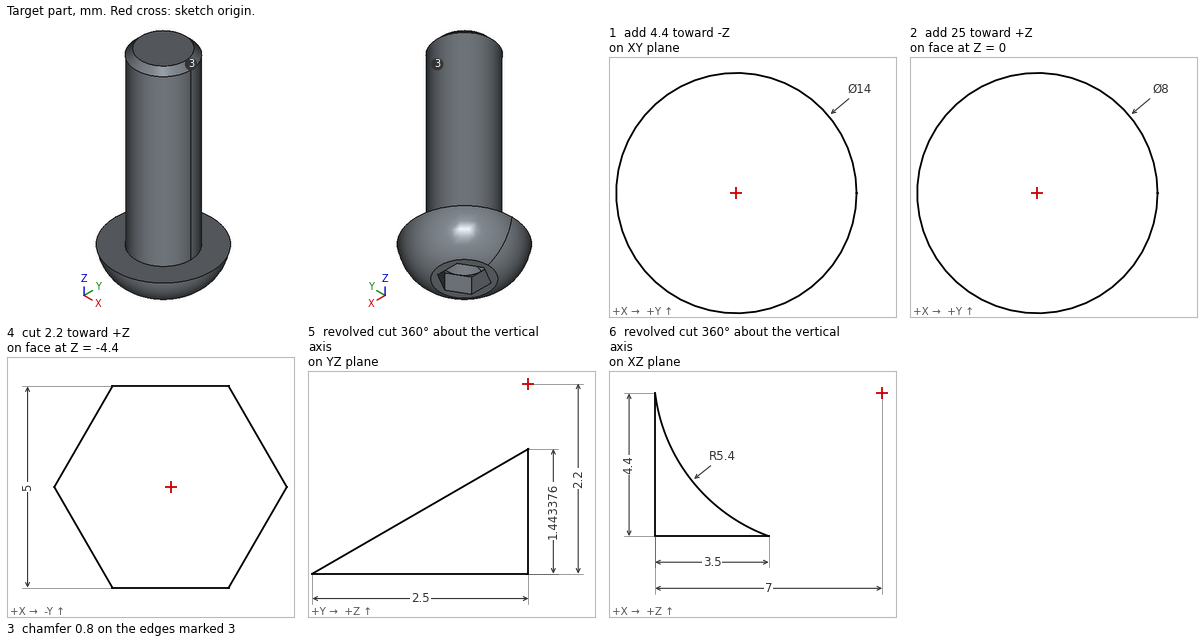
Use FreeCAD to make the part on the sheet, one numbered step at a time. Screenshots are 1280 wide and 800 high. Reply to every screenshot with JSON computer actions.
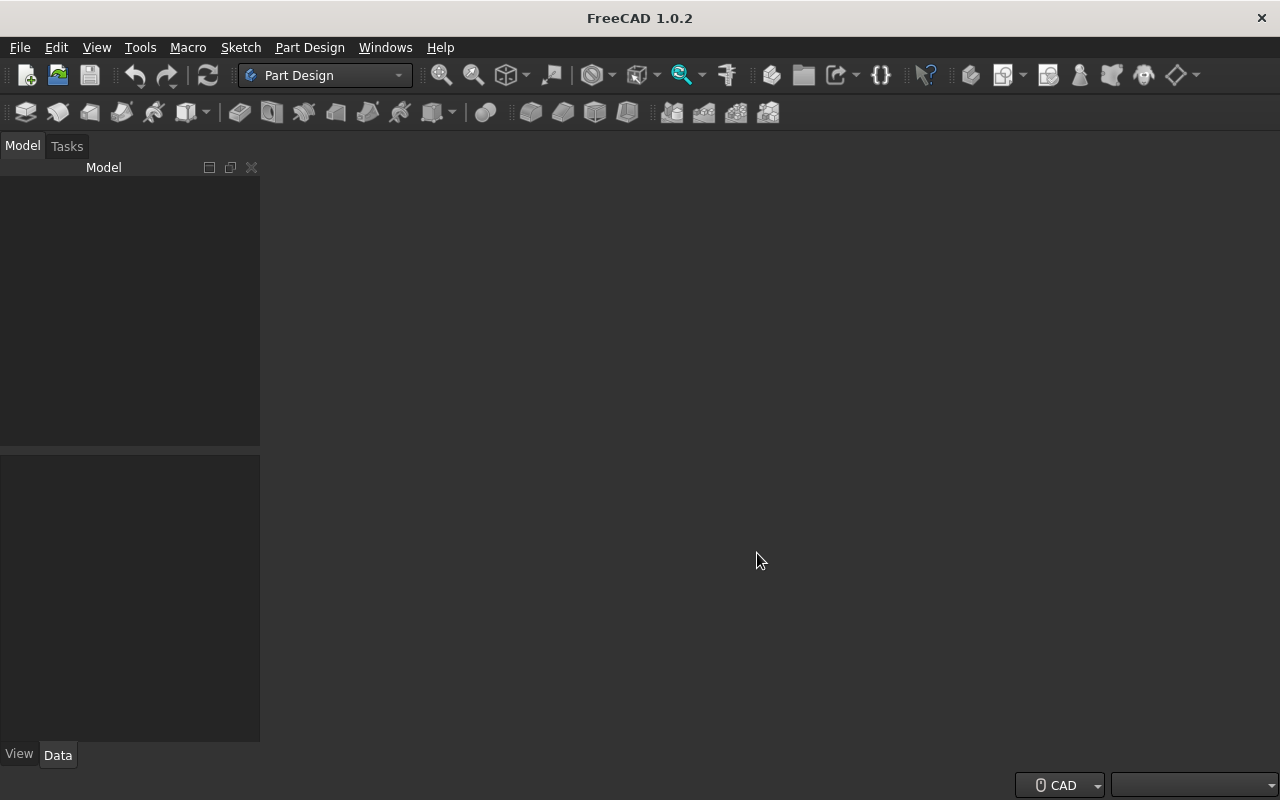
{"action": "key", "text": "ctrl+n"}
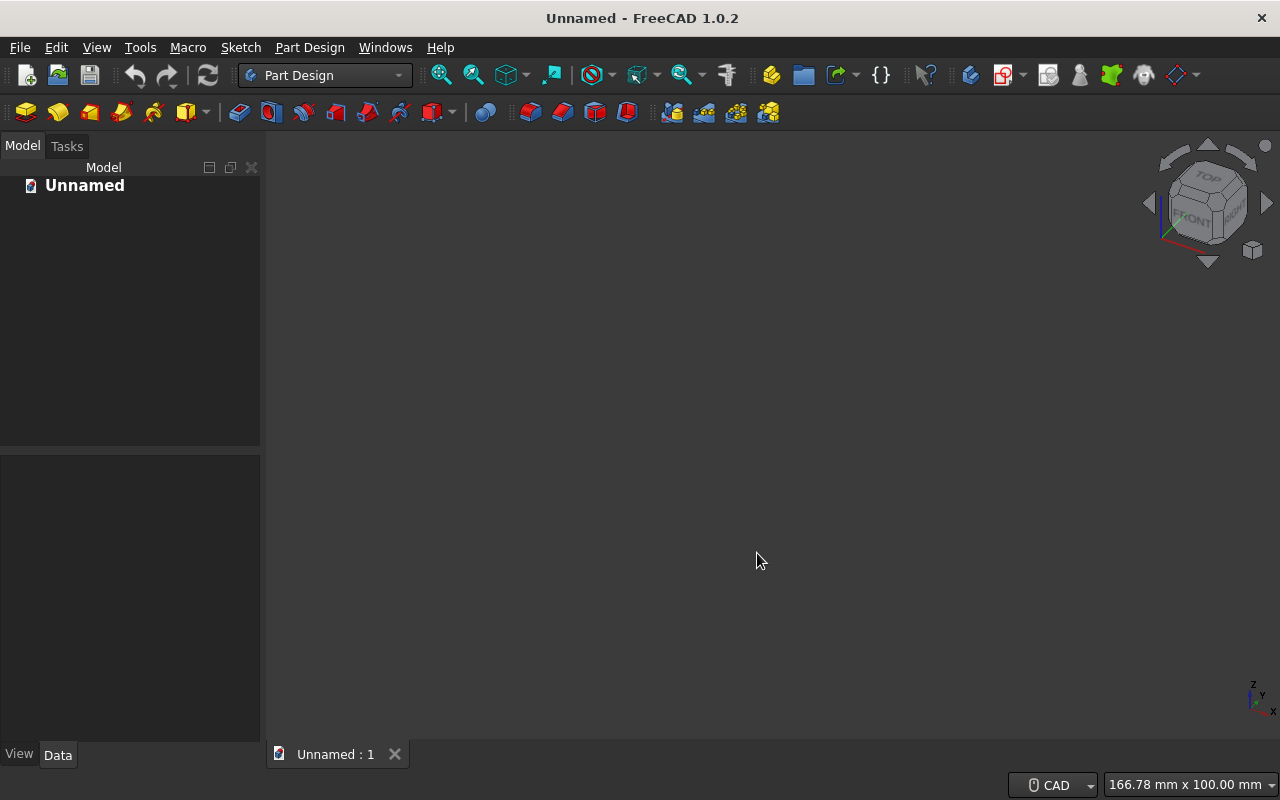
{"action": "left_click", "coordinate": [1004, 76]}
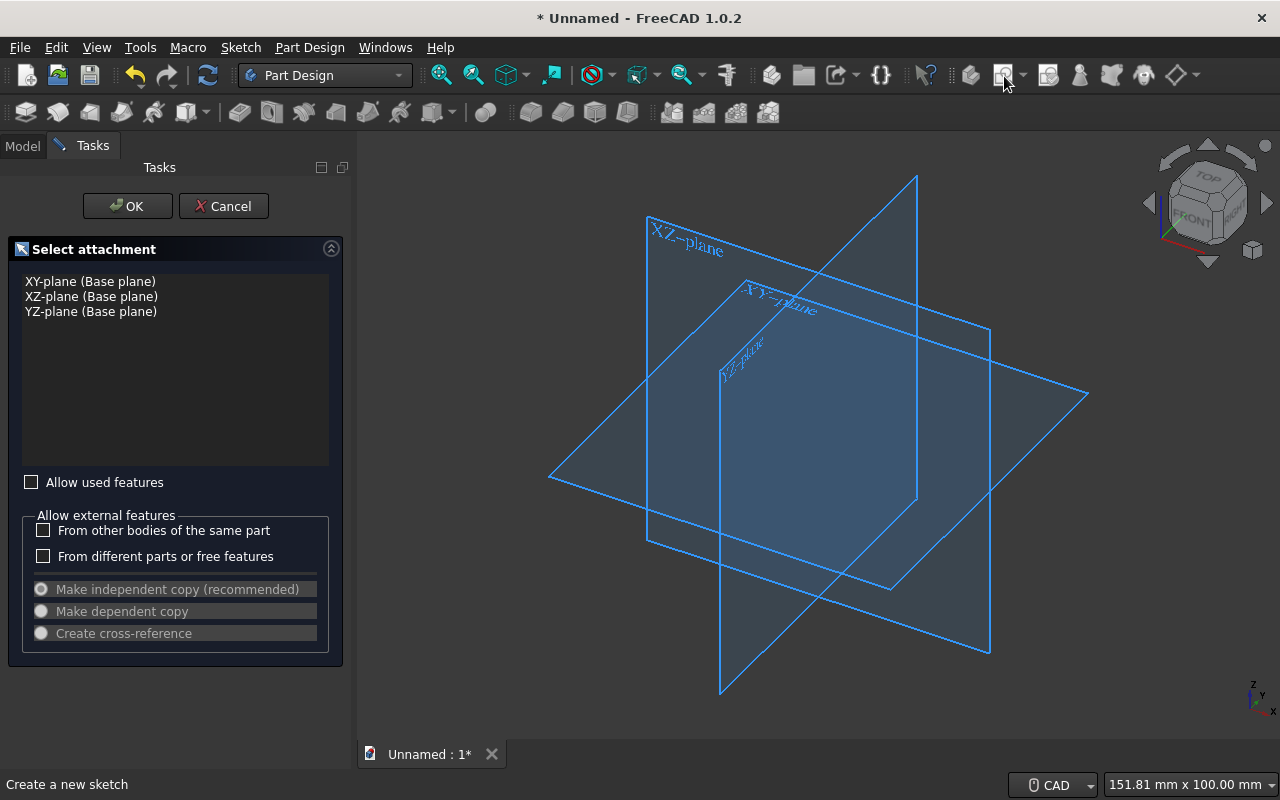
{"action": "left_click", "coordinate": [82, 282]}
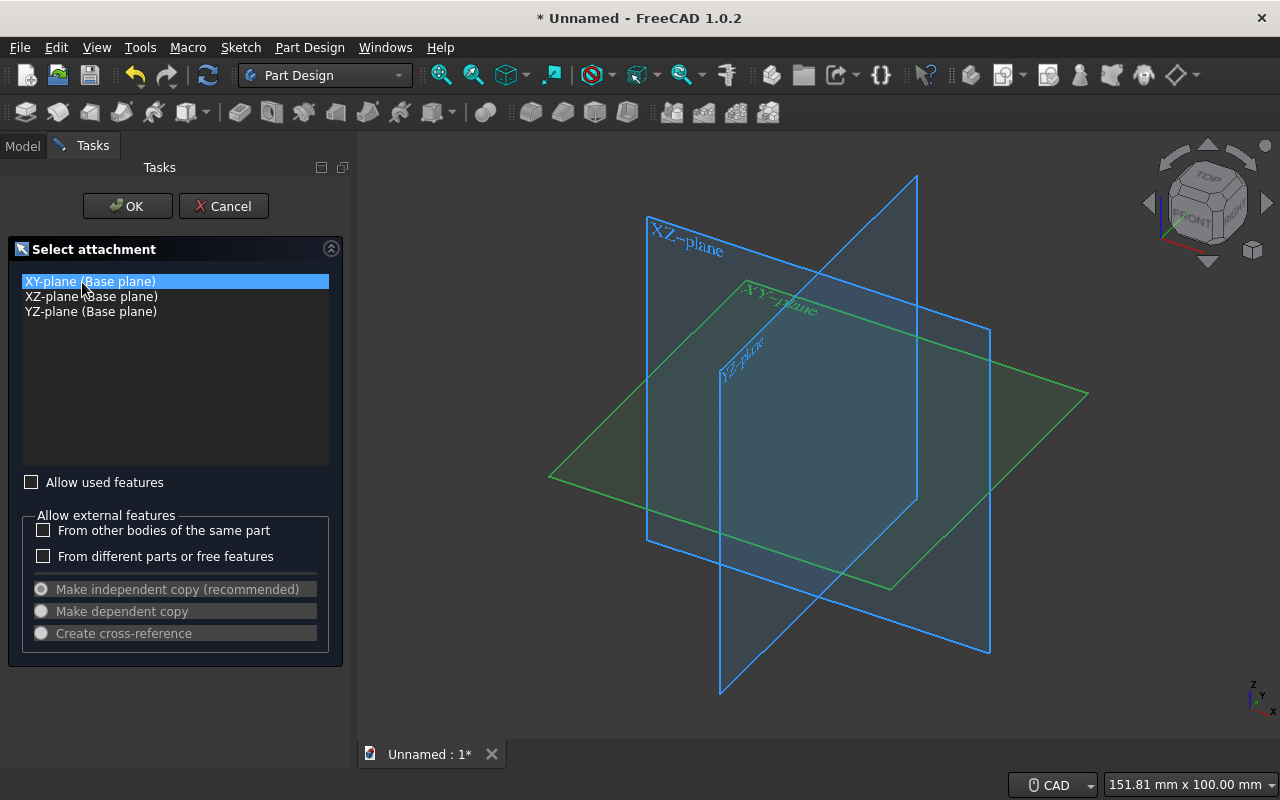
{"action": "left_click", "coordinate": [128, 206]}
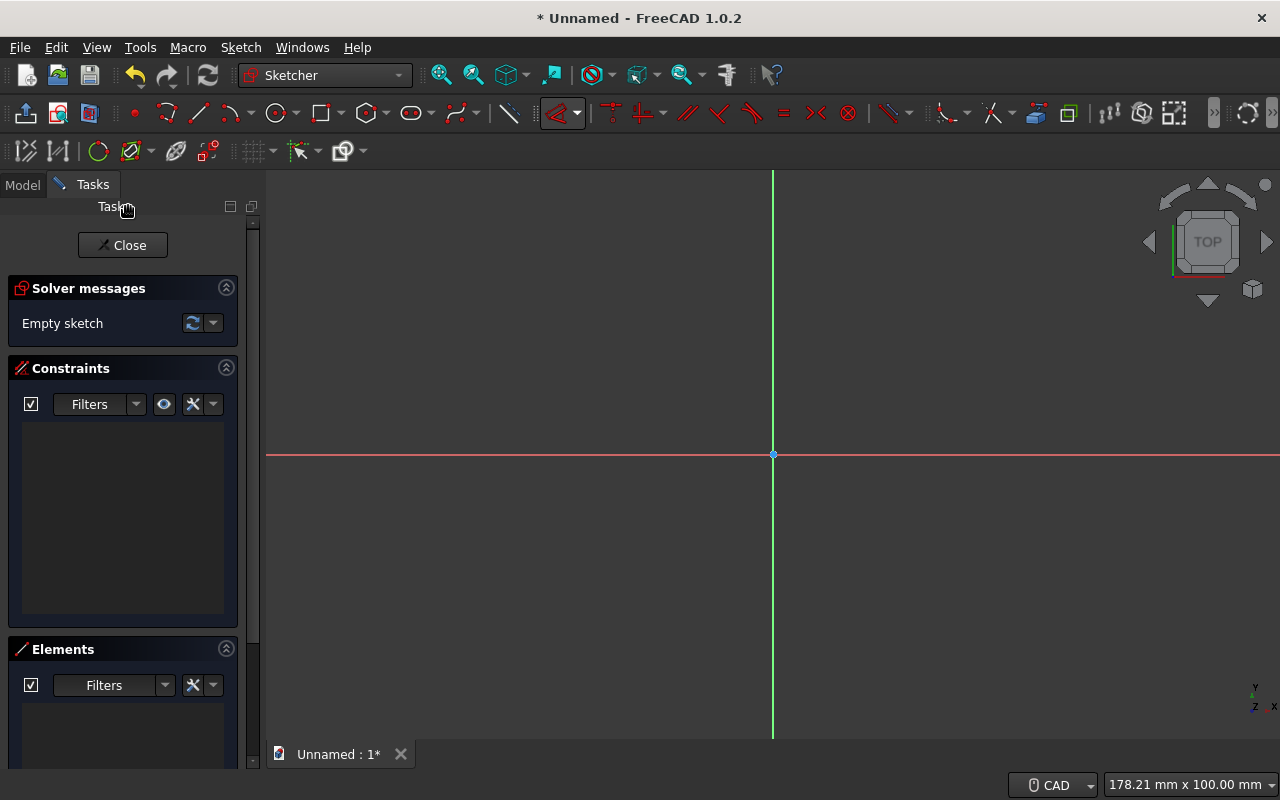
{"action": "scroll", "coordinate": [790, 454], "scroll_direction": "up", "scroll_amount": 8}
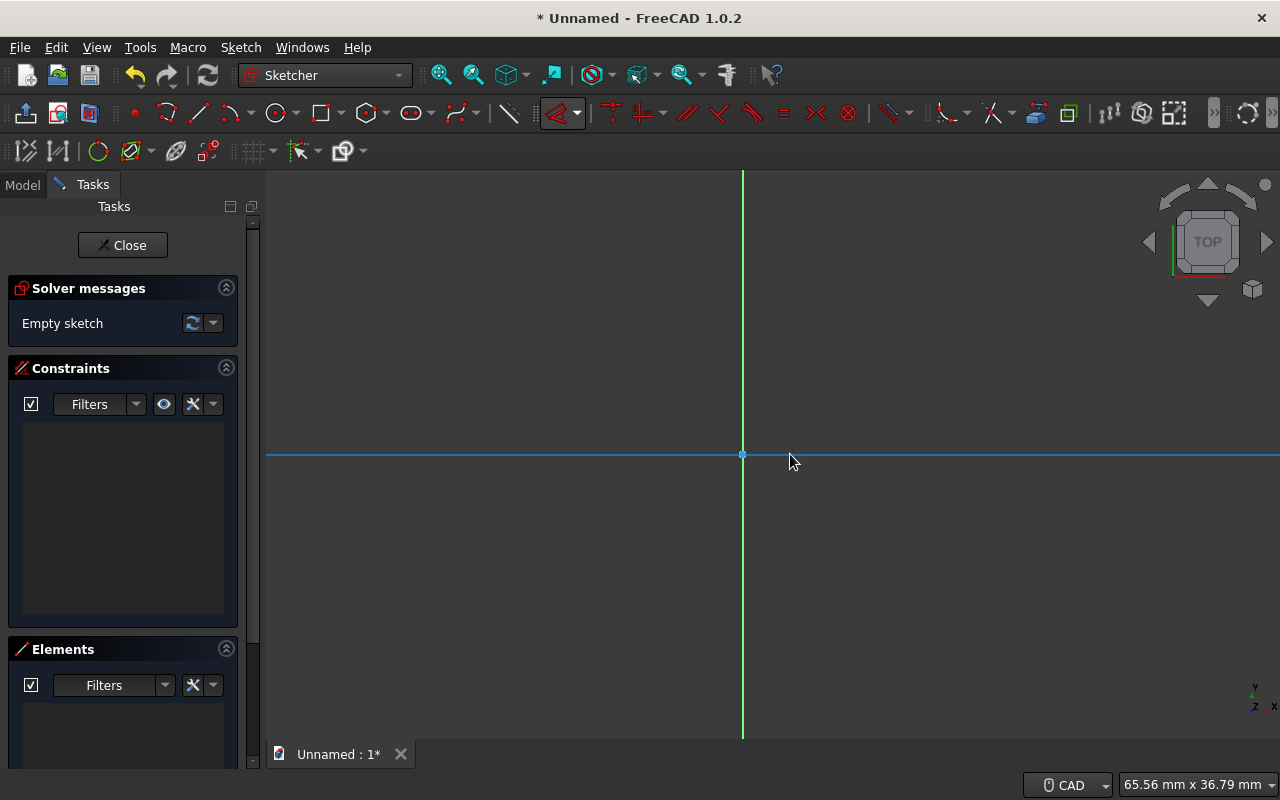
{"action": "left_click", "coordinate": [276, 114]}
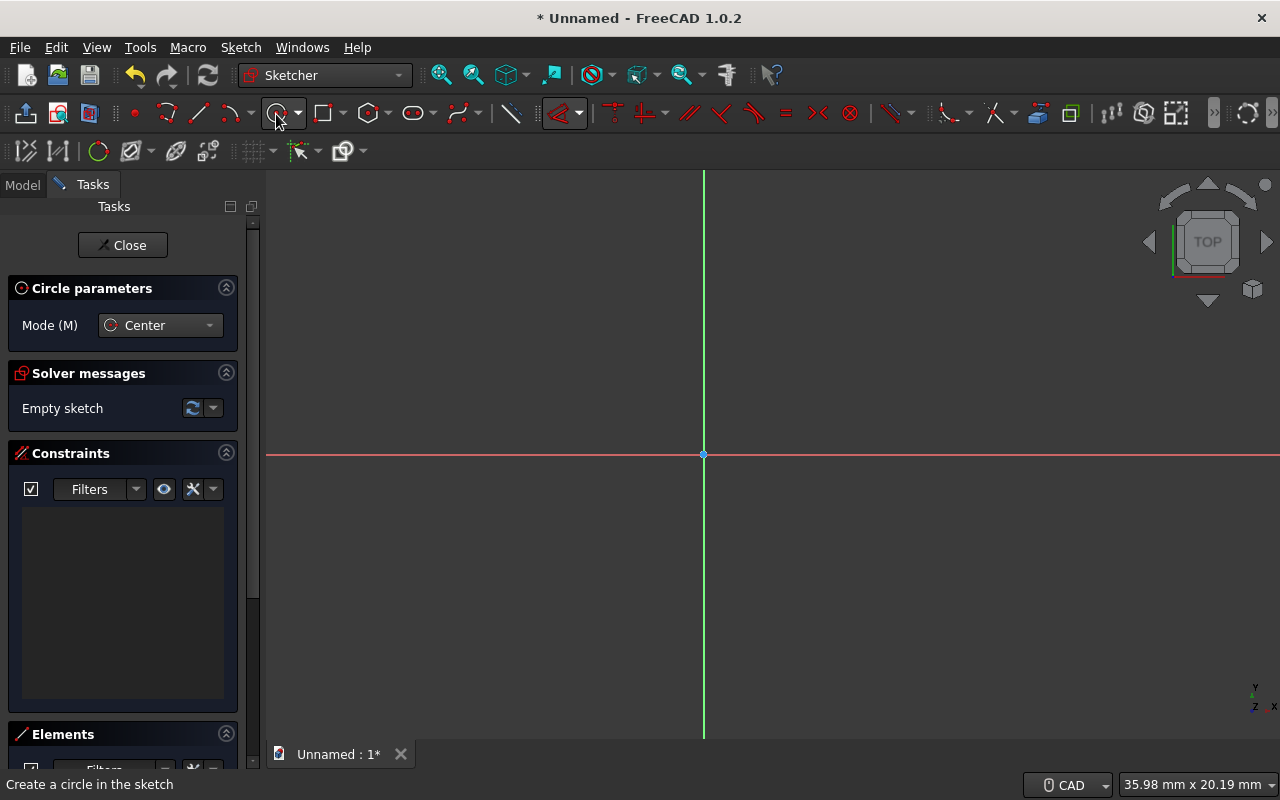
{"action": "left_click", "coordinate": [704, 454]}
{"action": "mouse_move", "coordinate": [843, 315]}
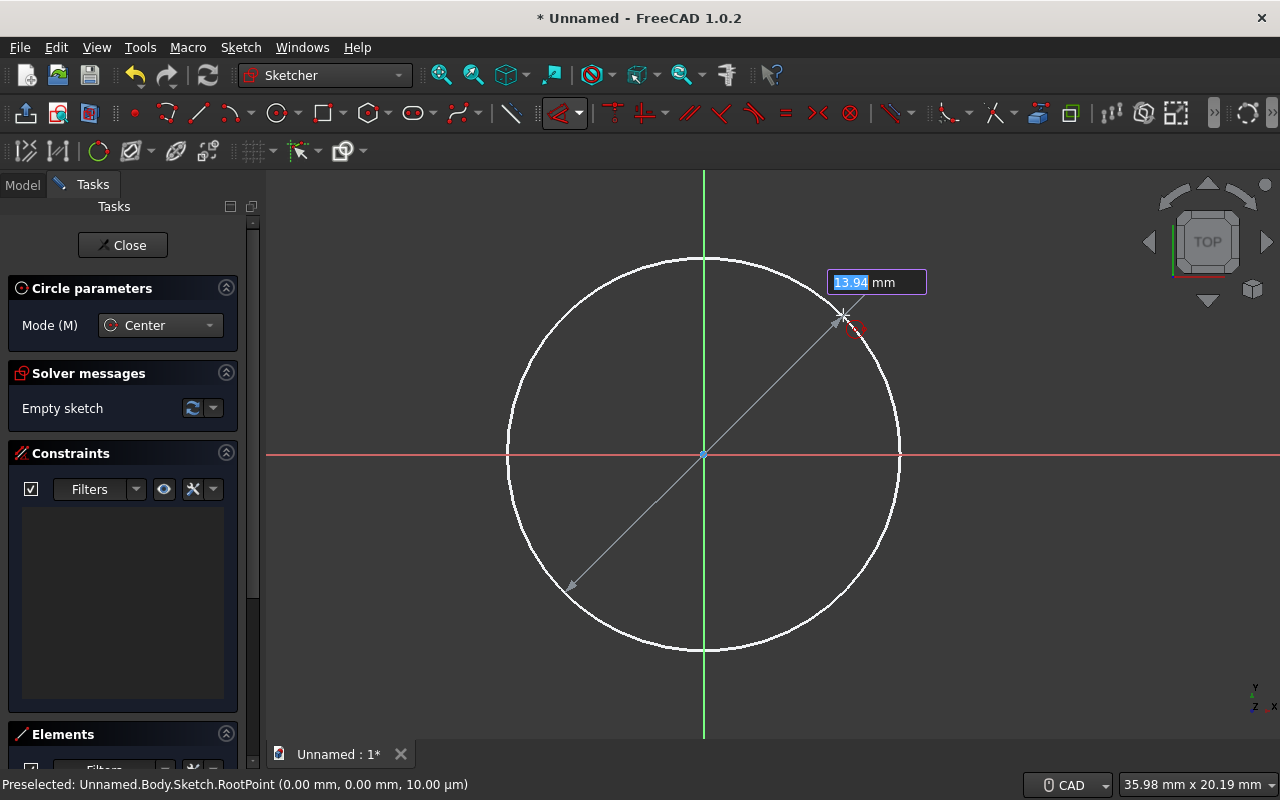
{"action": "type", "text": "14"}
{"action": "key", "text": "Return"}
{"action": "key", "text": "Escape"}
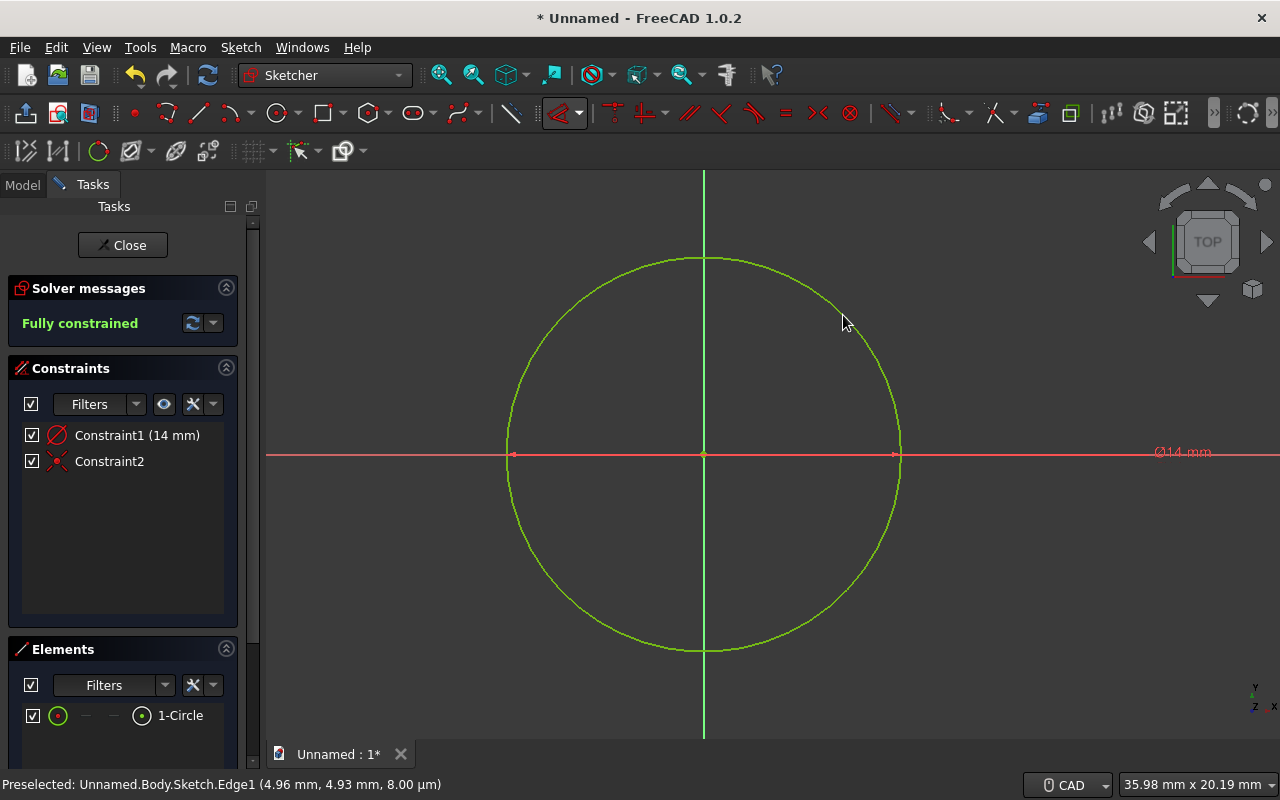
{"action": "left_click", "coordinate": [123, 245]}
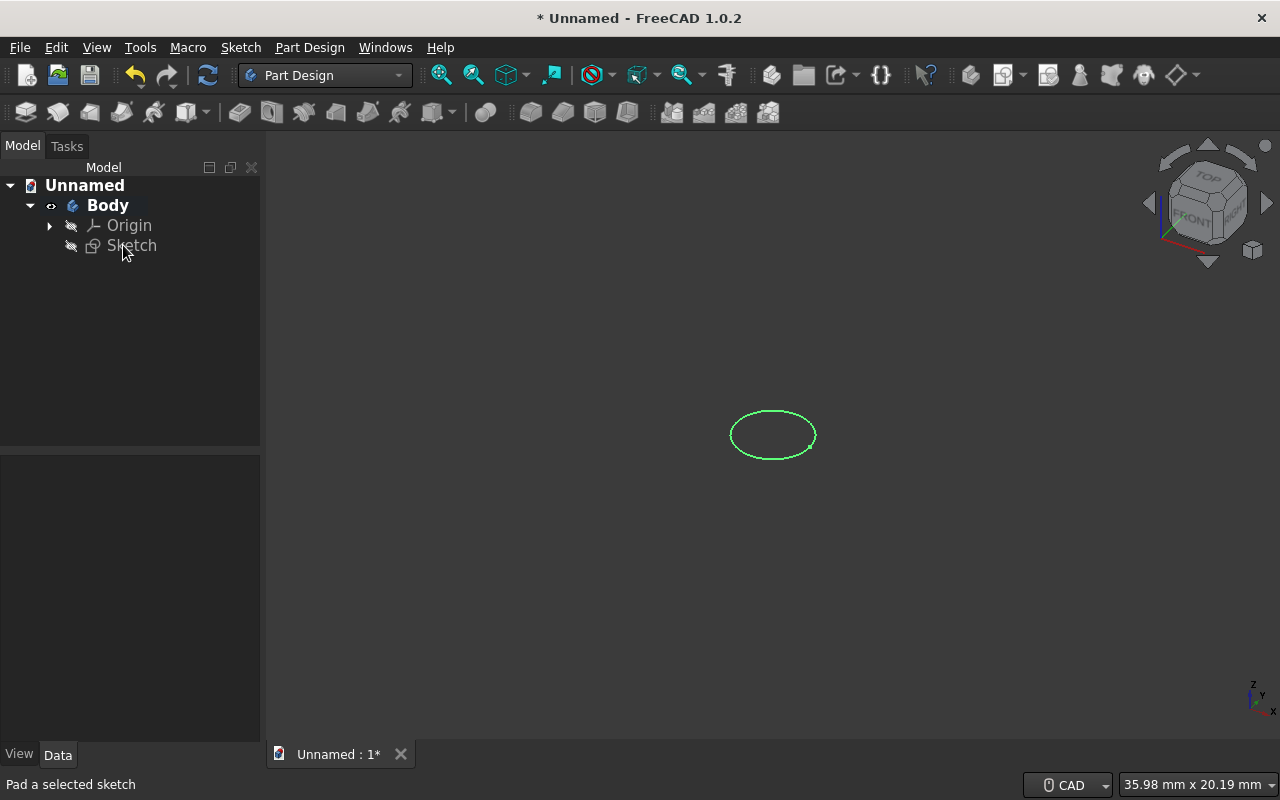
{"action": "left_click", "coordinate": [26, 112]}